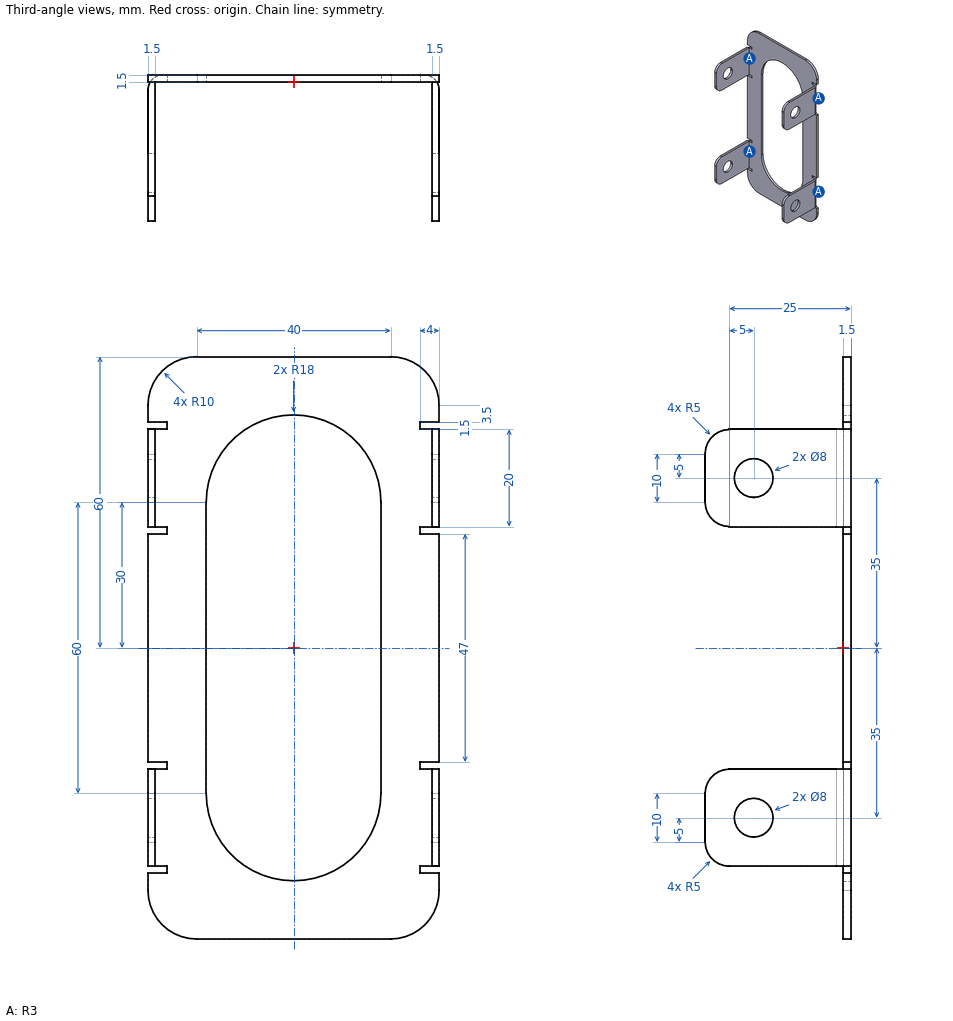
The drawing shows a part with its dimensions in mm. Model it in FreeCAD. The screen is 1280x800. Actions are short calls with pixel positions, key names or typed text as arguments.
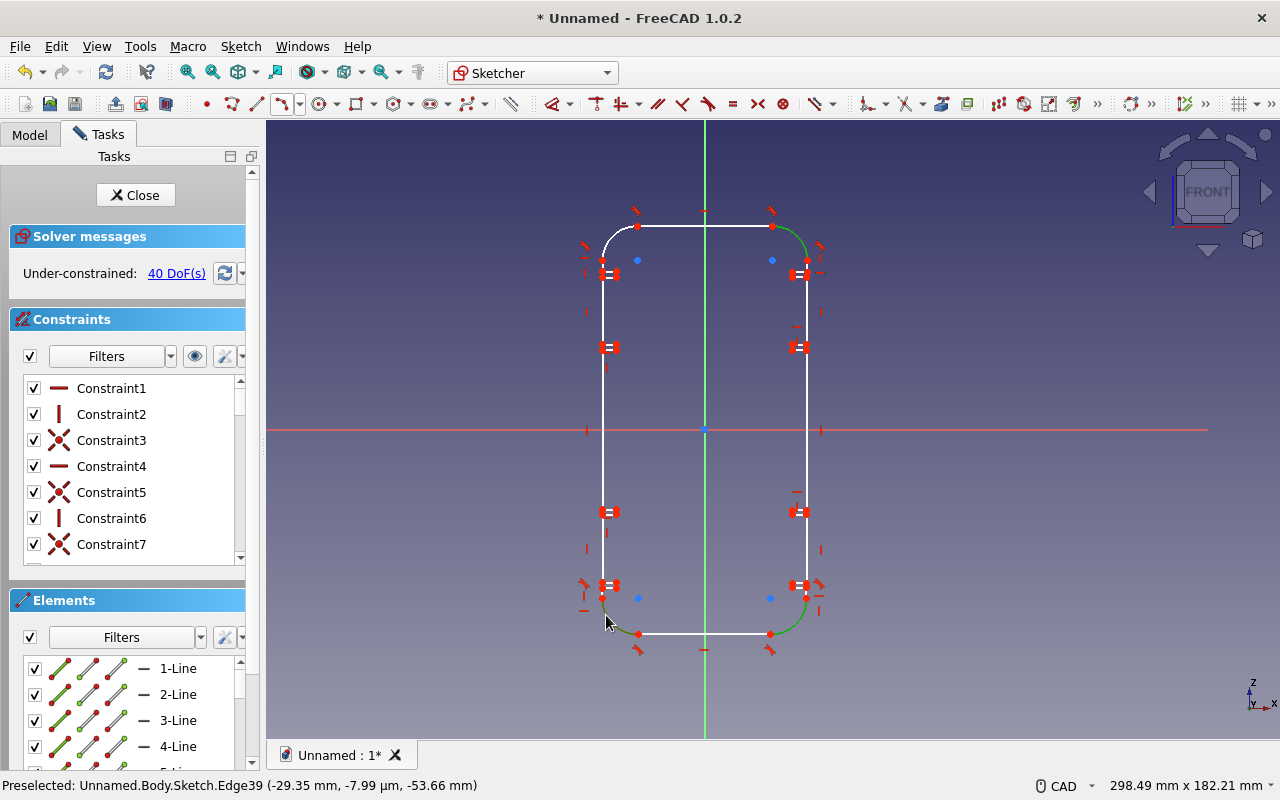
click(621, 230)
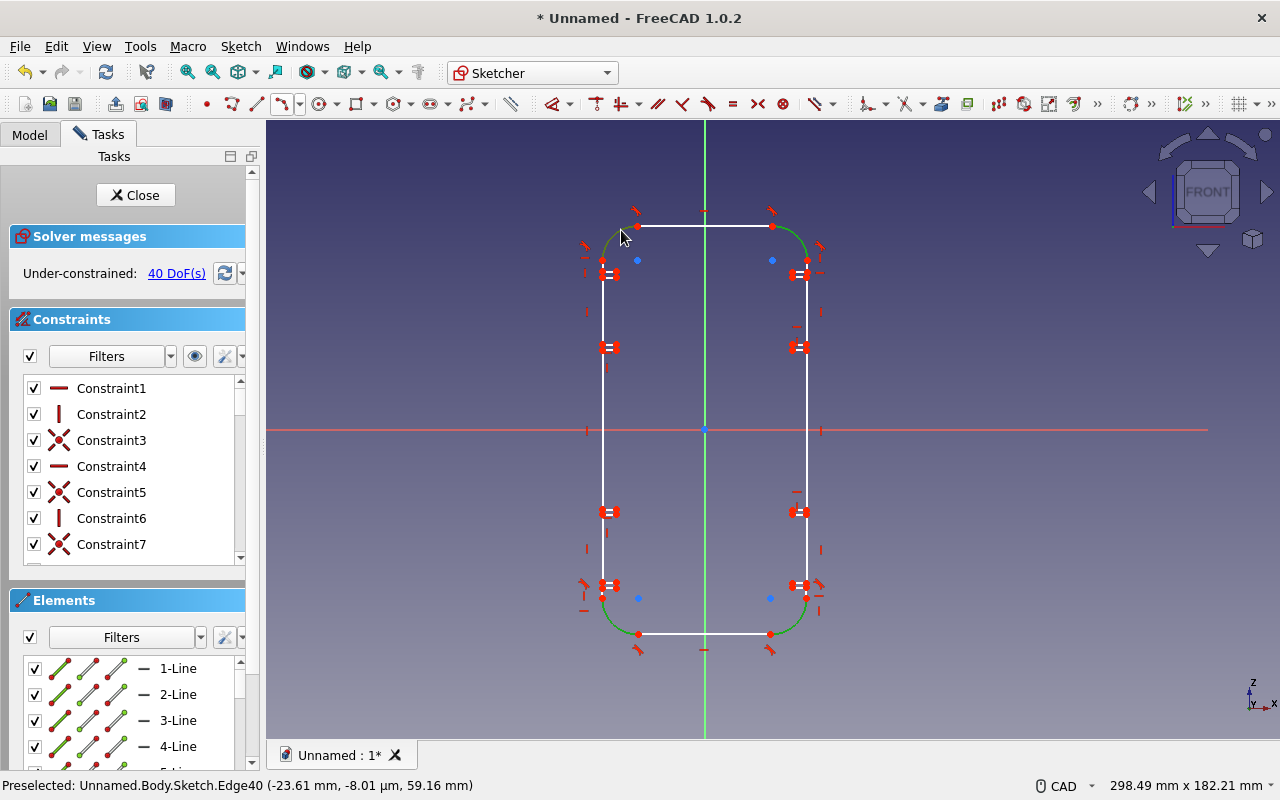
click(733, 104)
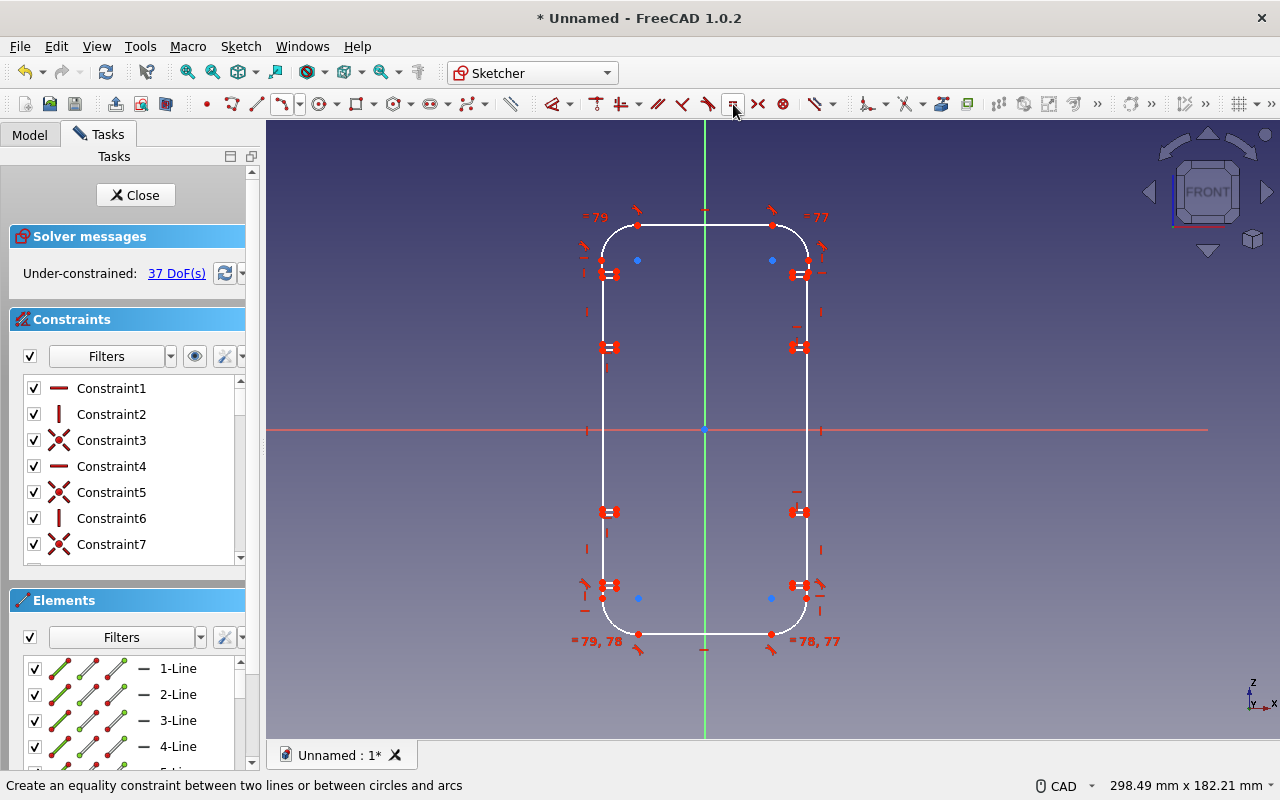
click(773, 261)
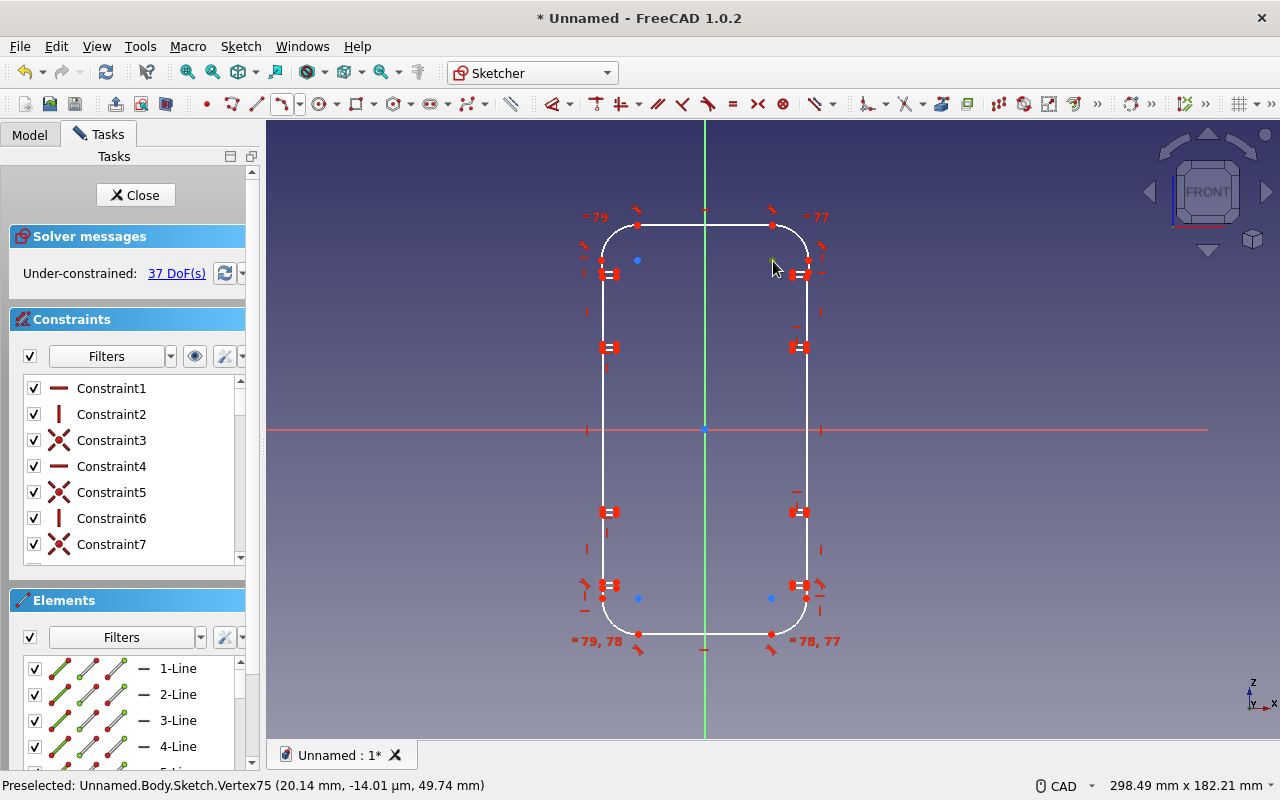
click(771, 599)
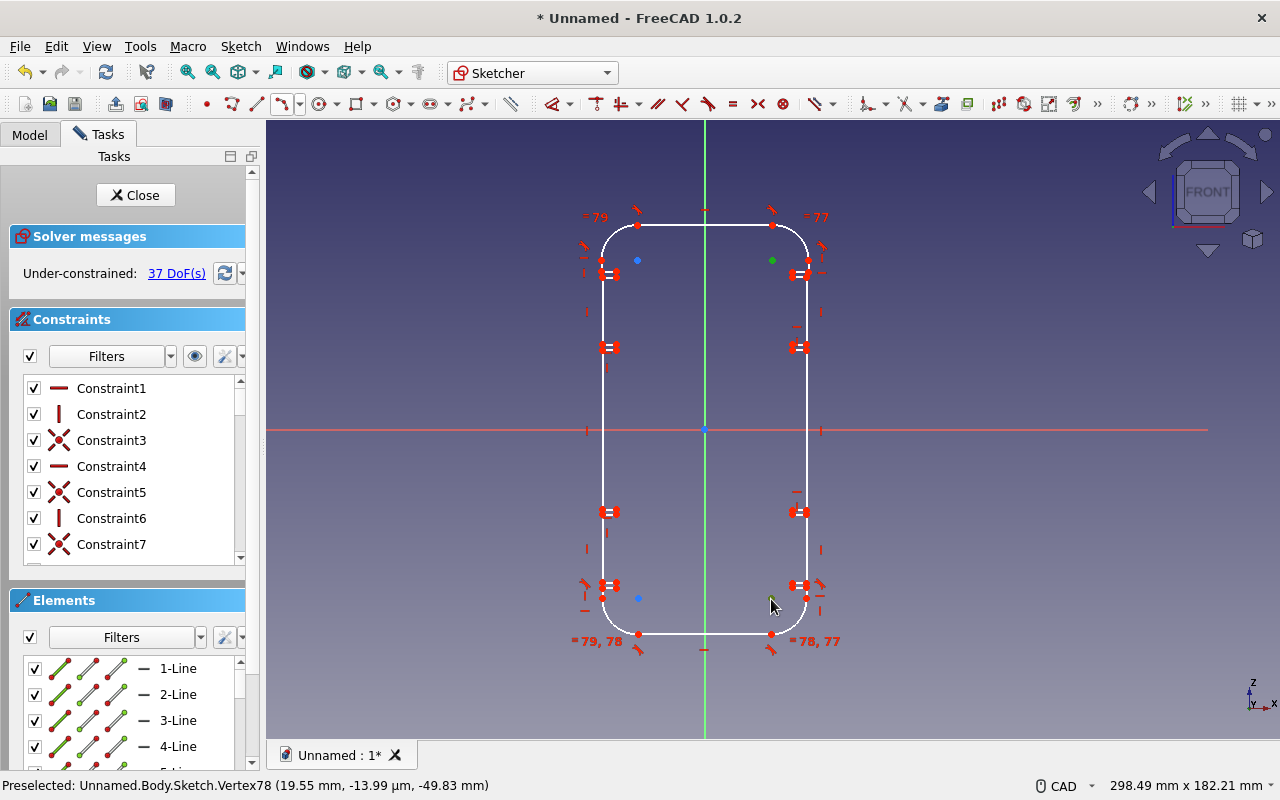
click(353, 430)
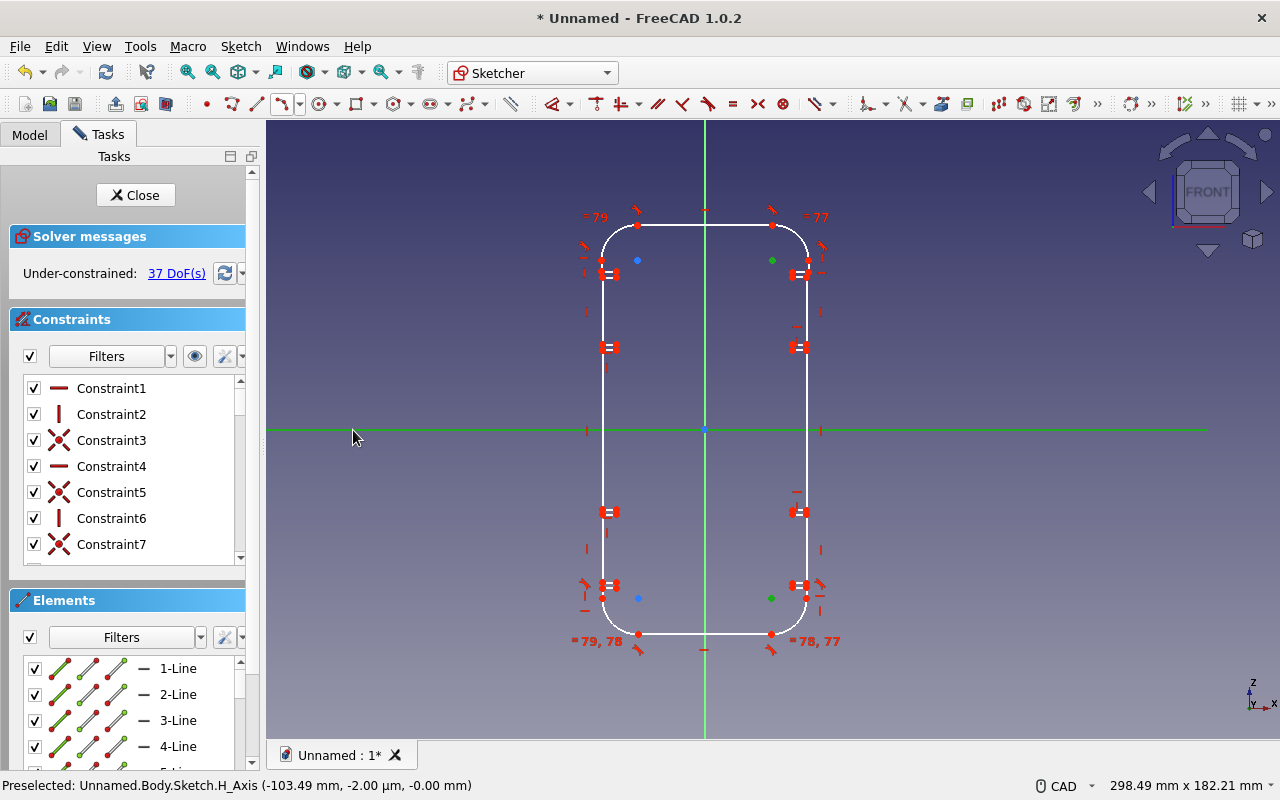
click(758, 104)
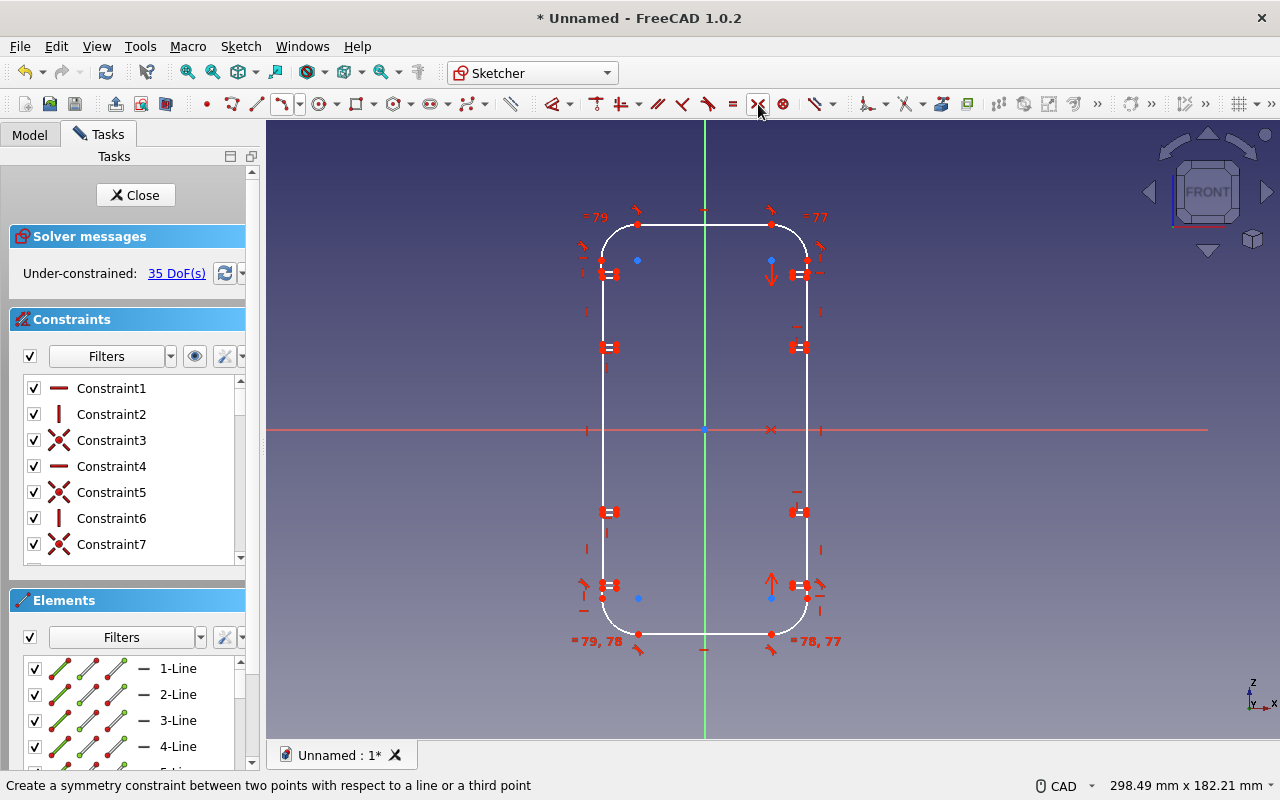
scroll(793, 350, up, 5)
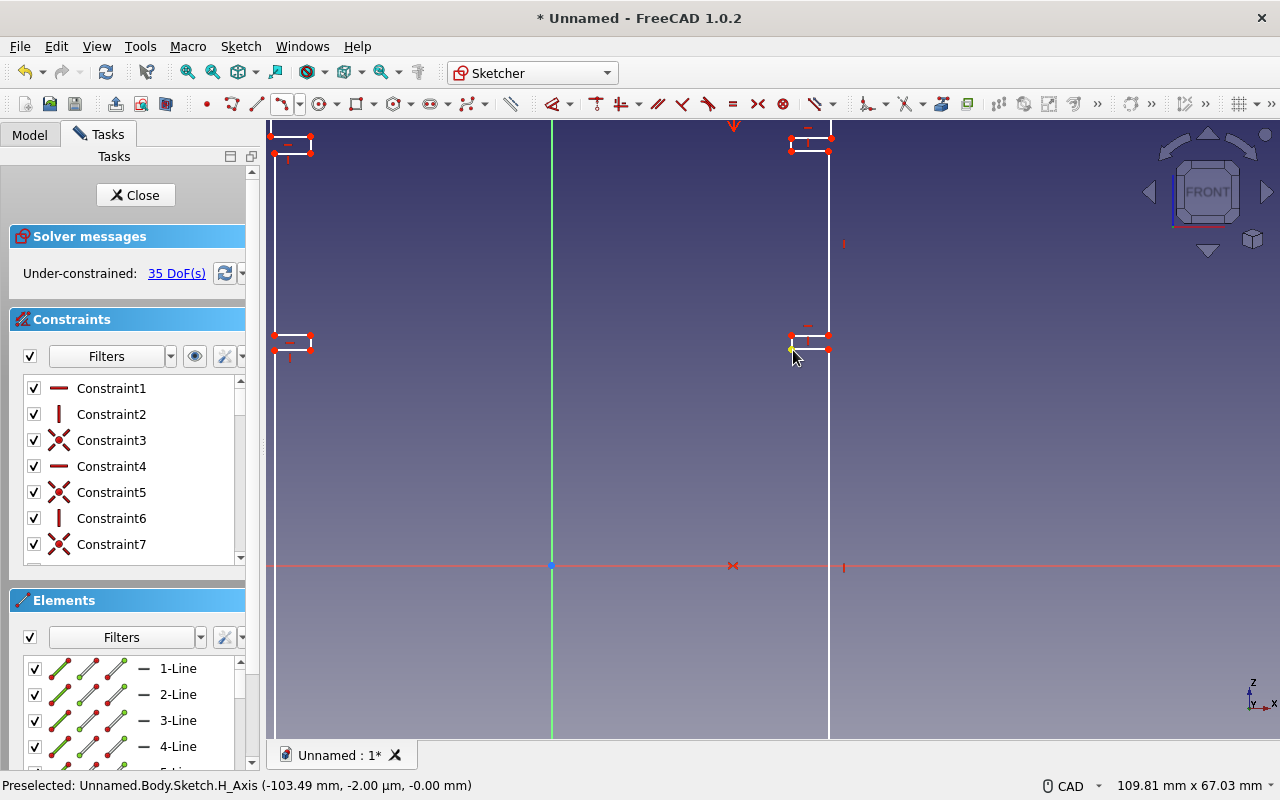
click(792, 349)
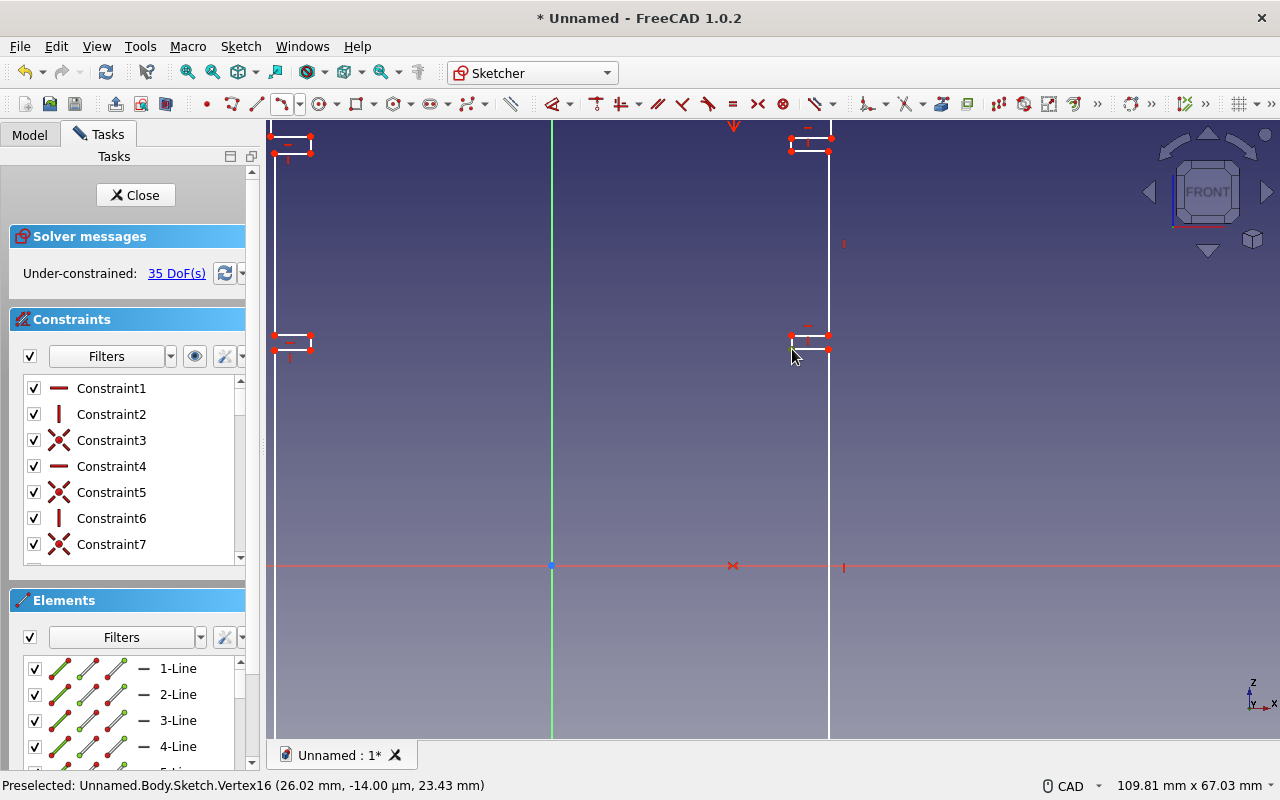
scroll(793, 350, down, 5)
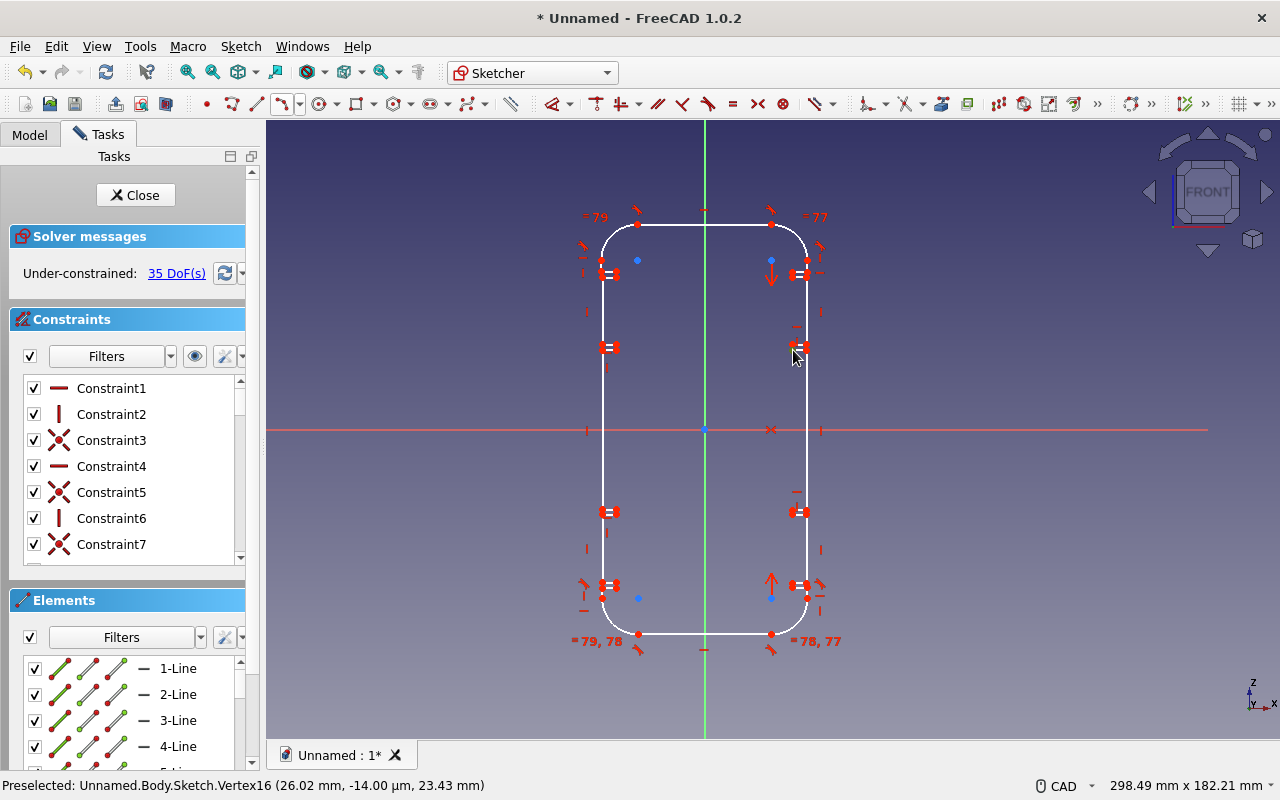
scroll(793, 510, up, 5)